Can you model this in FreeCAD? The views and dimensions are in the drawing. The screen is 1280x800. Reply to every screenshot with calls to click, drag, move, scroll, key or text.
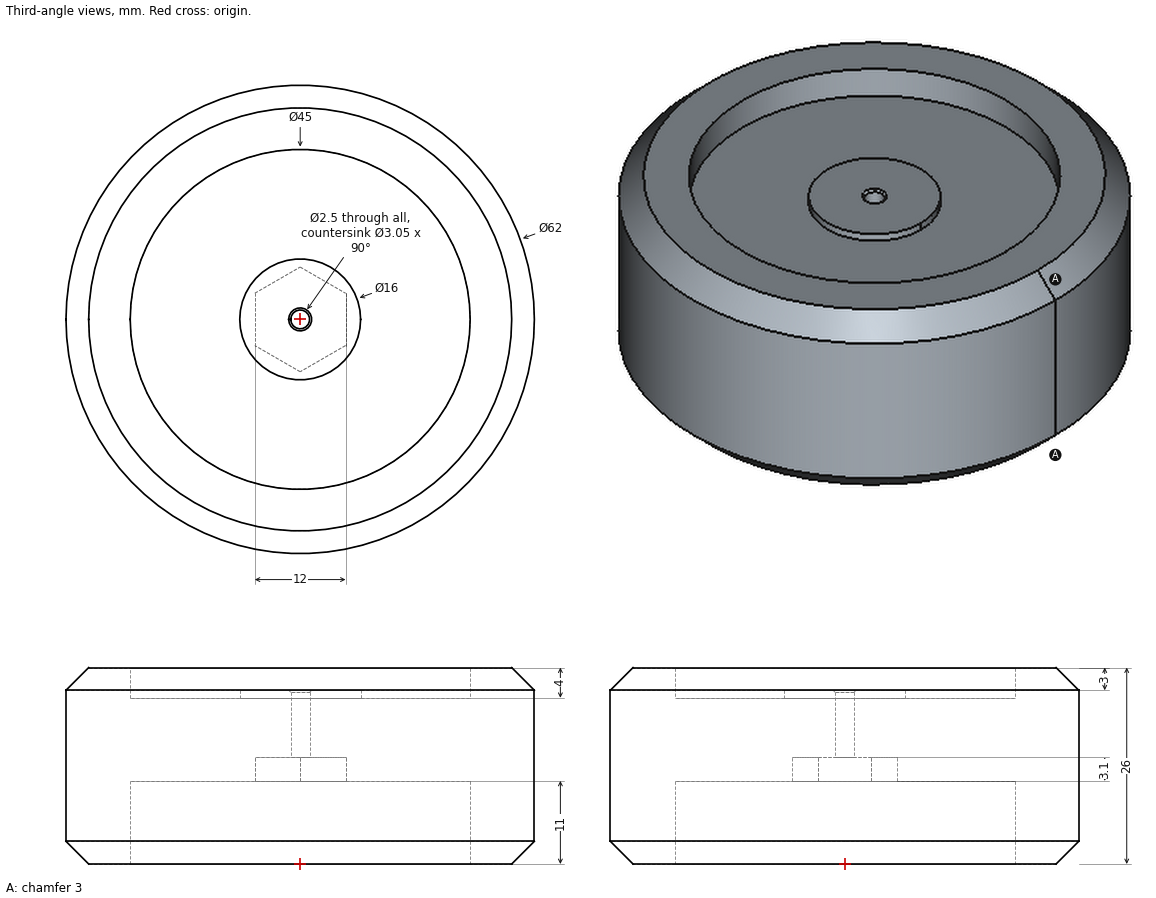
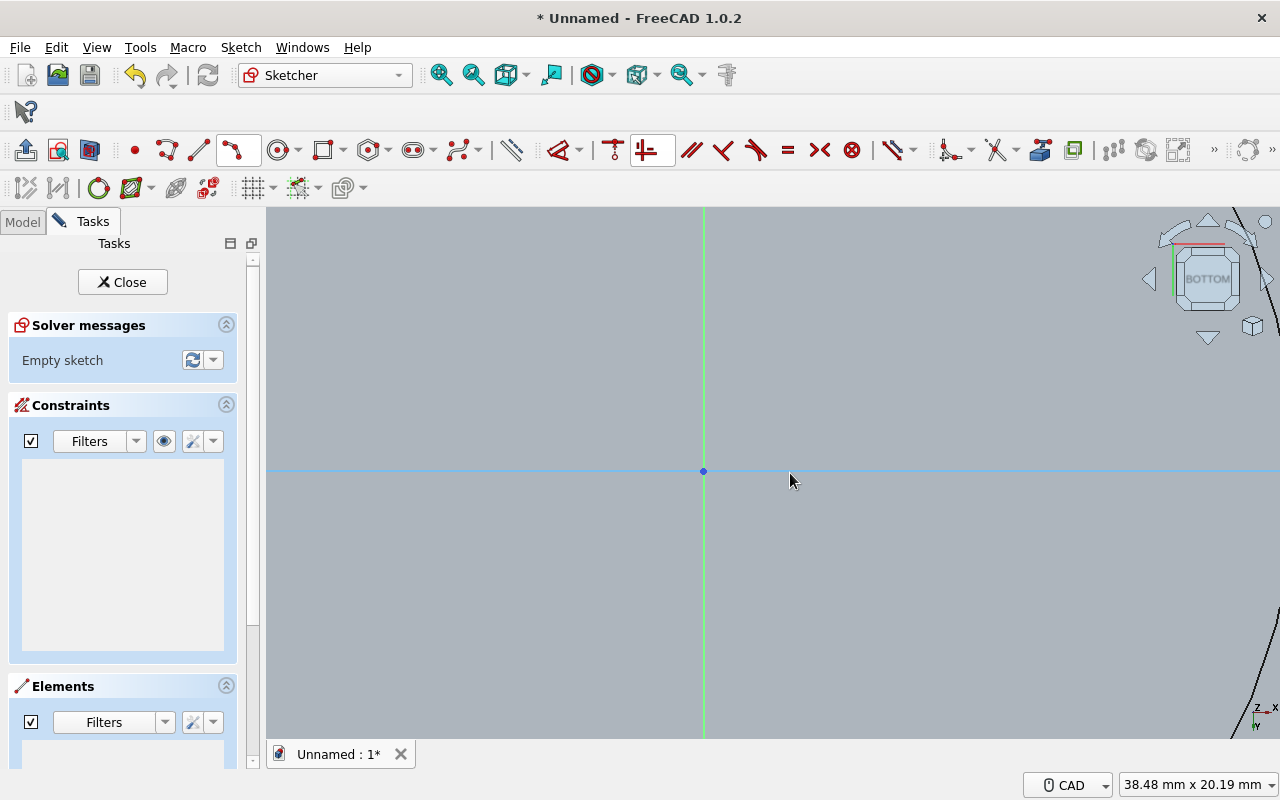
click(368, 150)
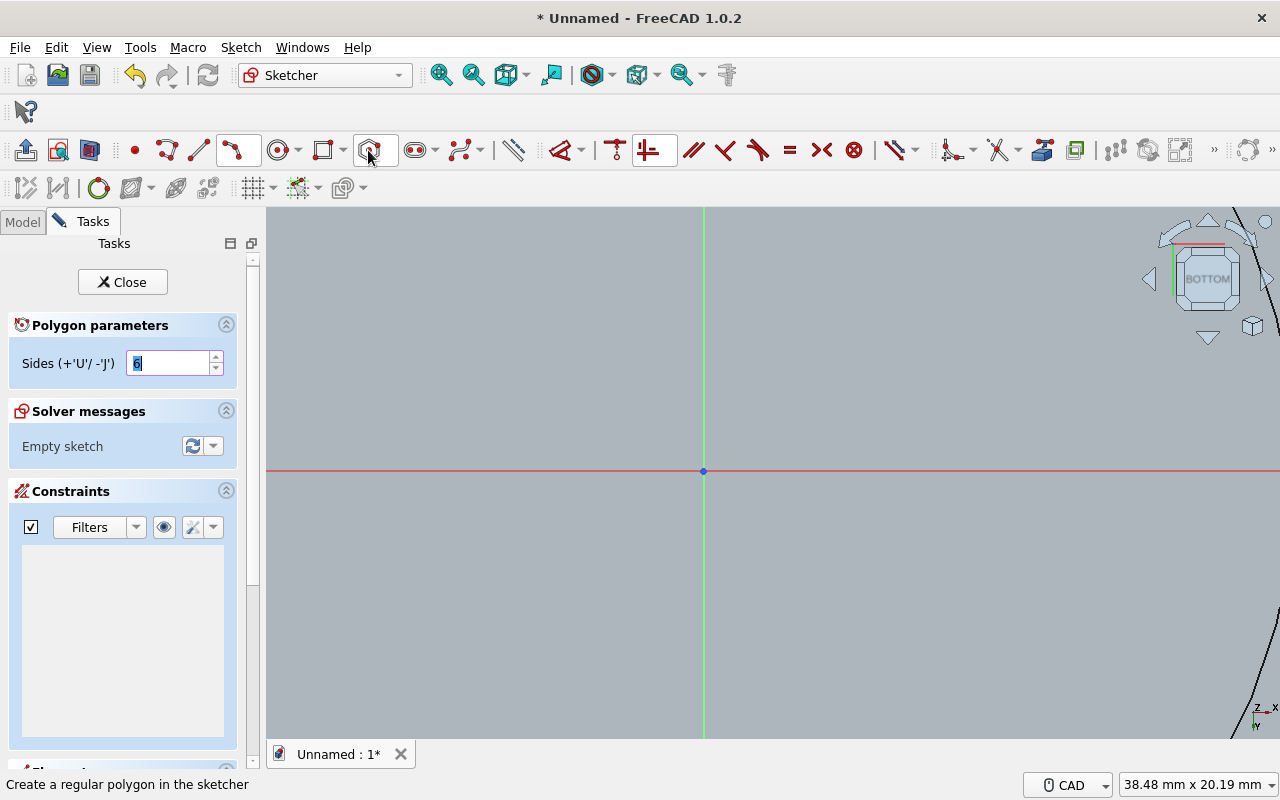
click(704, 471)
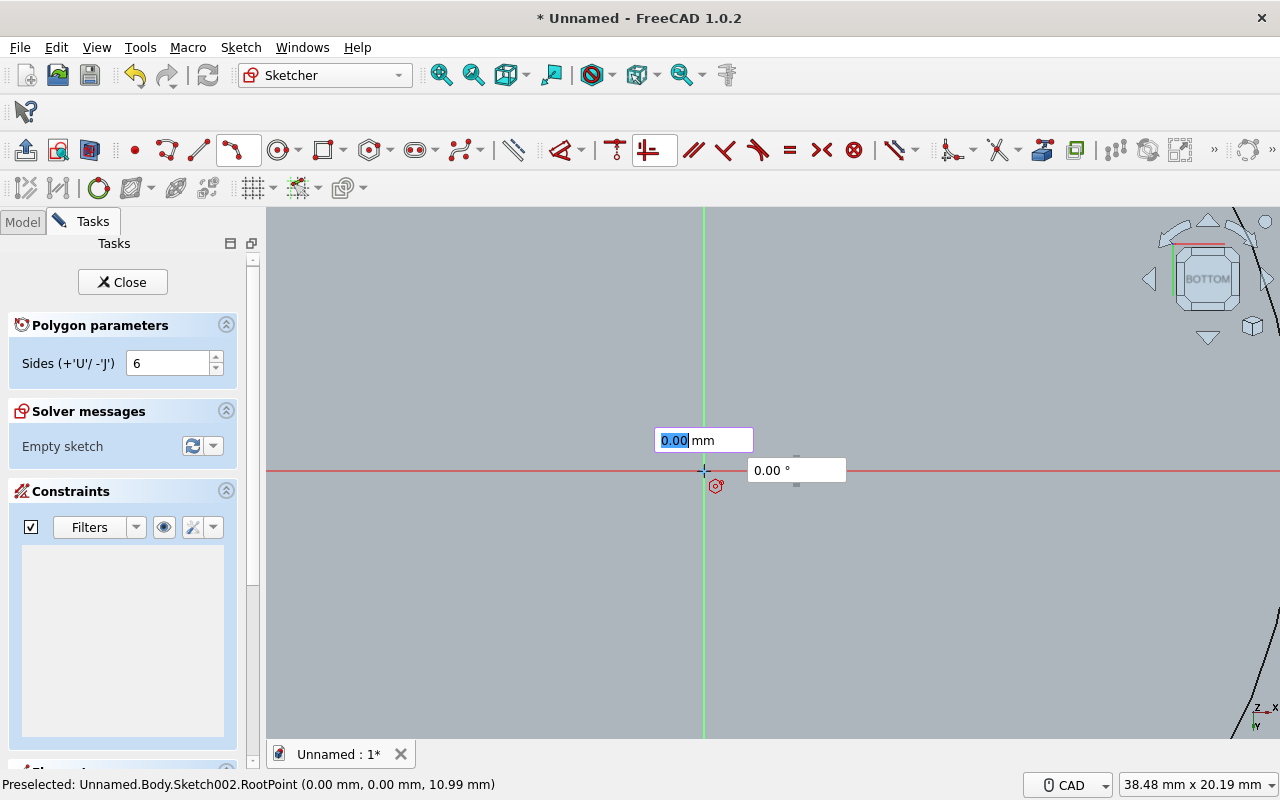
click(704, 654)
right_click(704, 654)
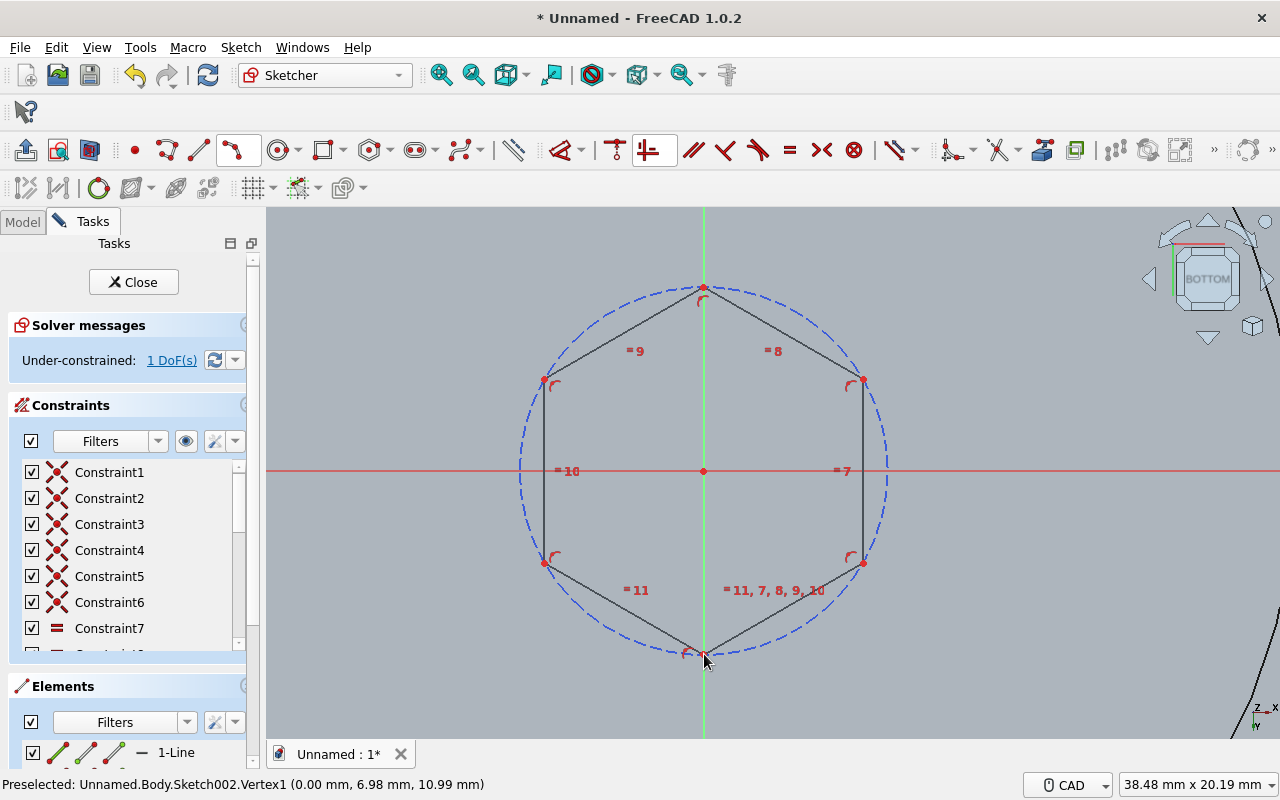
key(d)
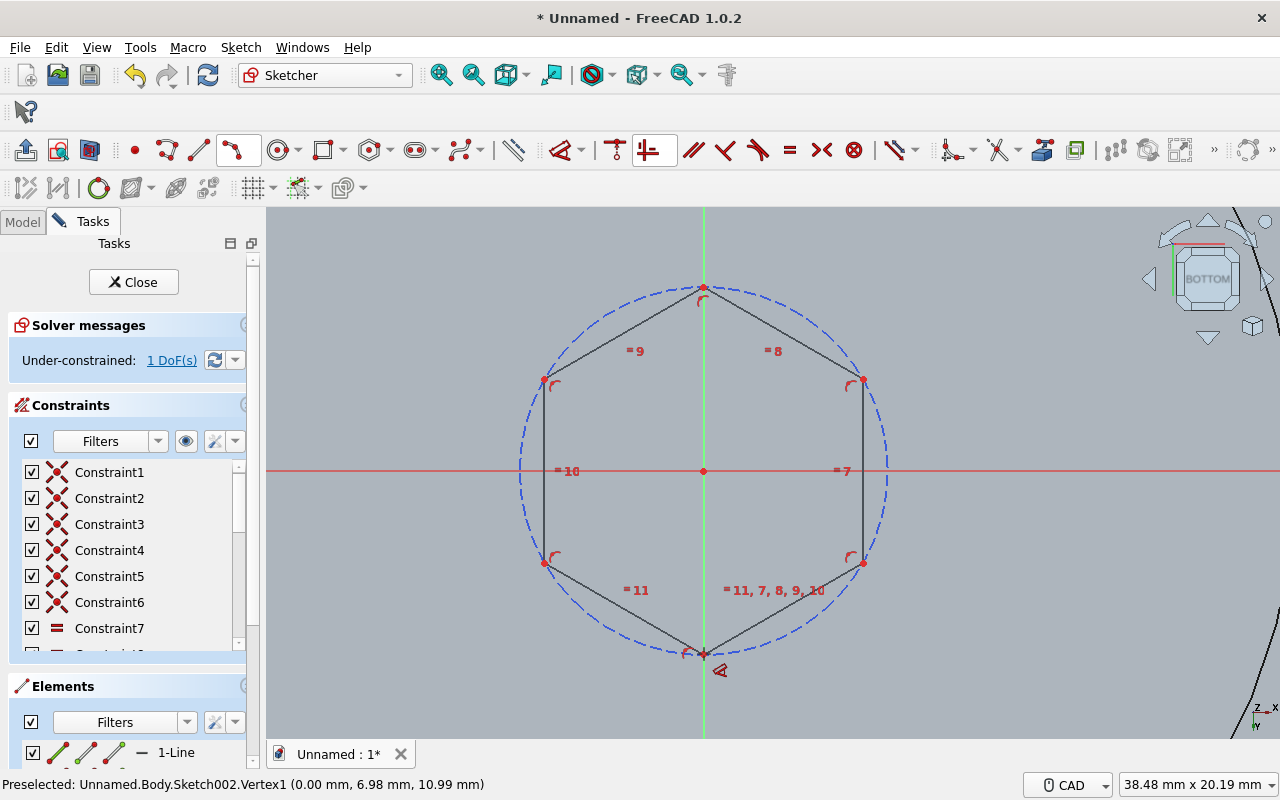
click(544, 379)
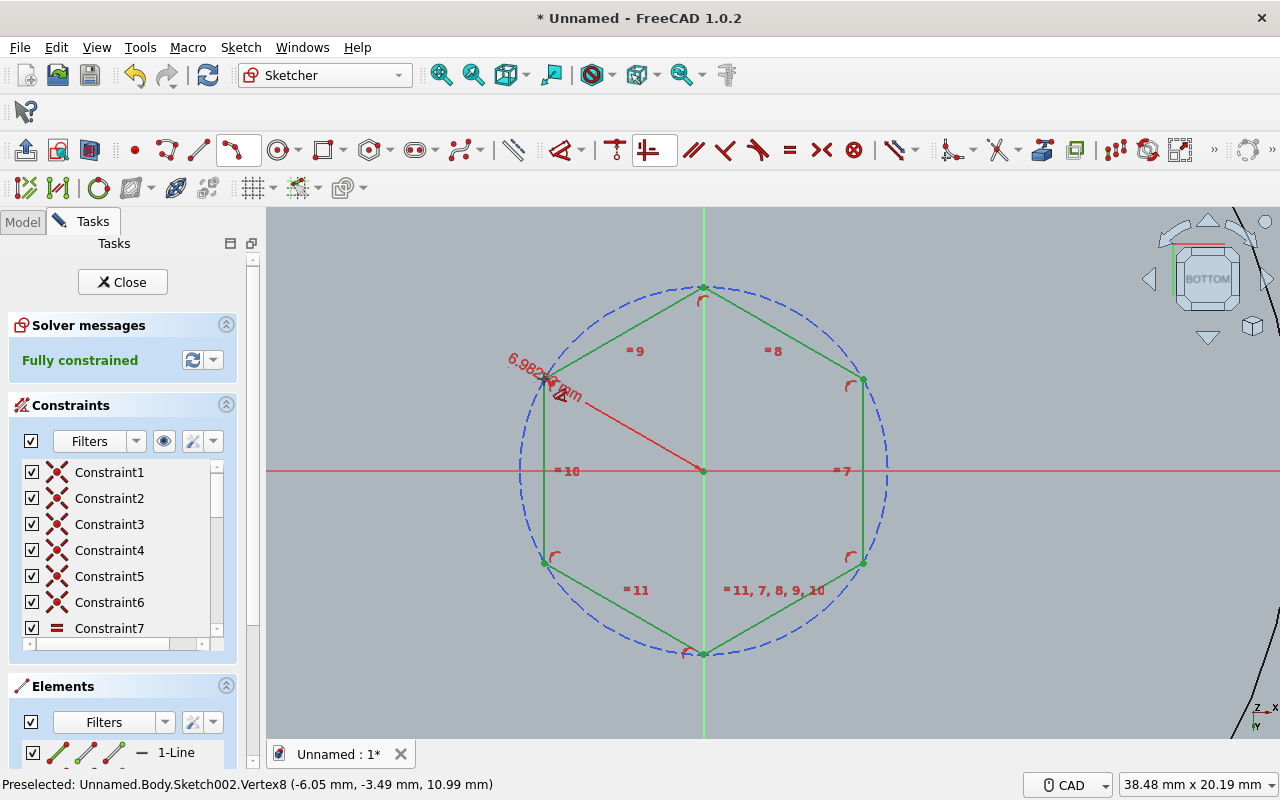
click(863, 563)
click(630, 597)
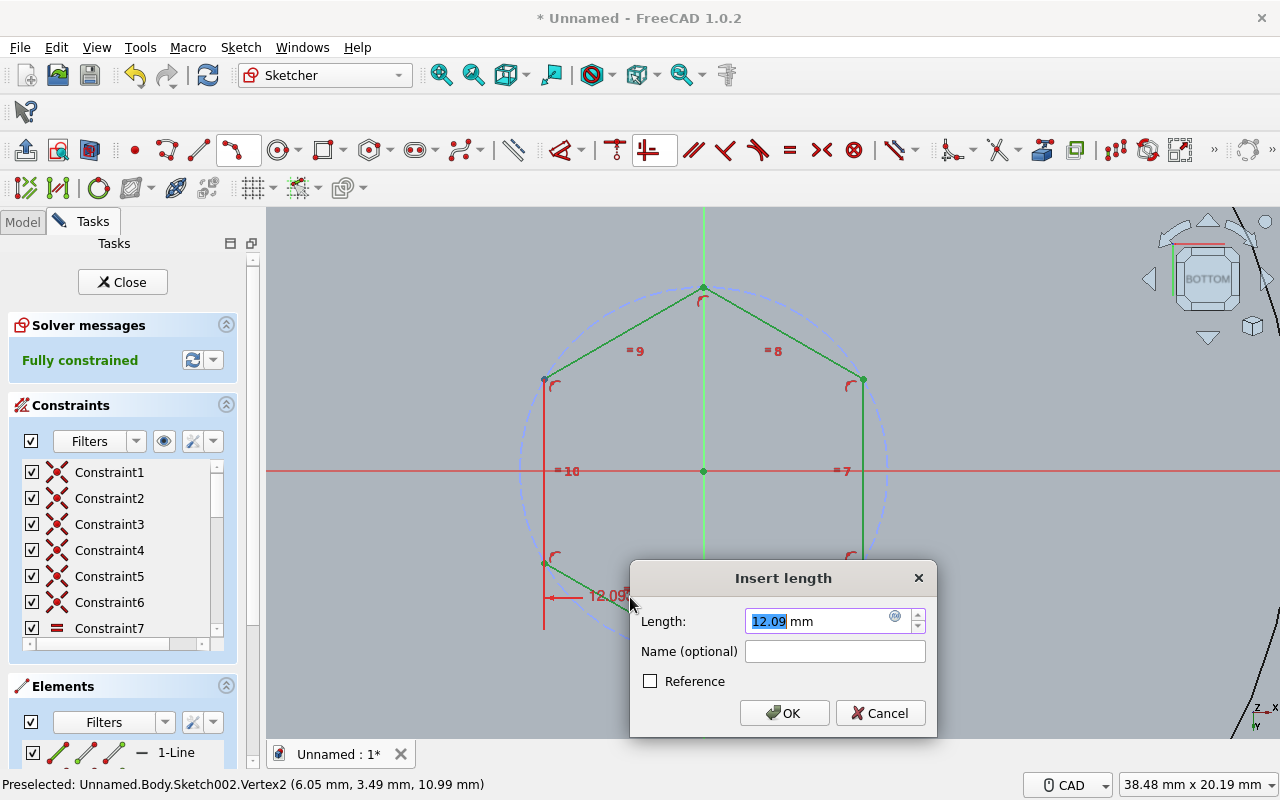
text(12)
key(Return)
key(Escape)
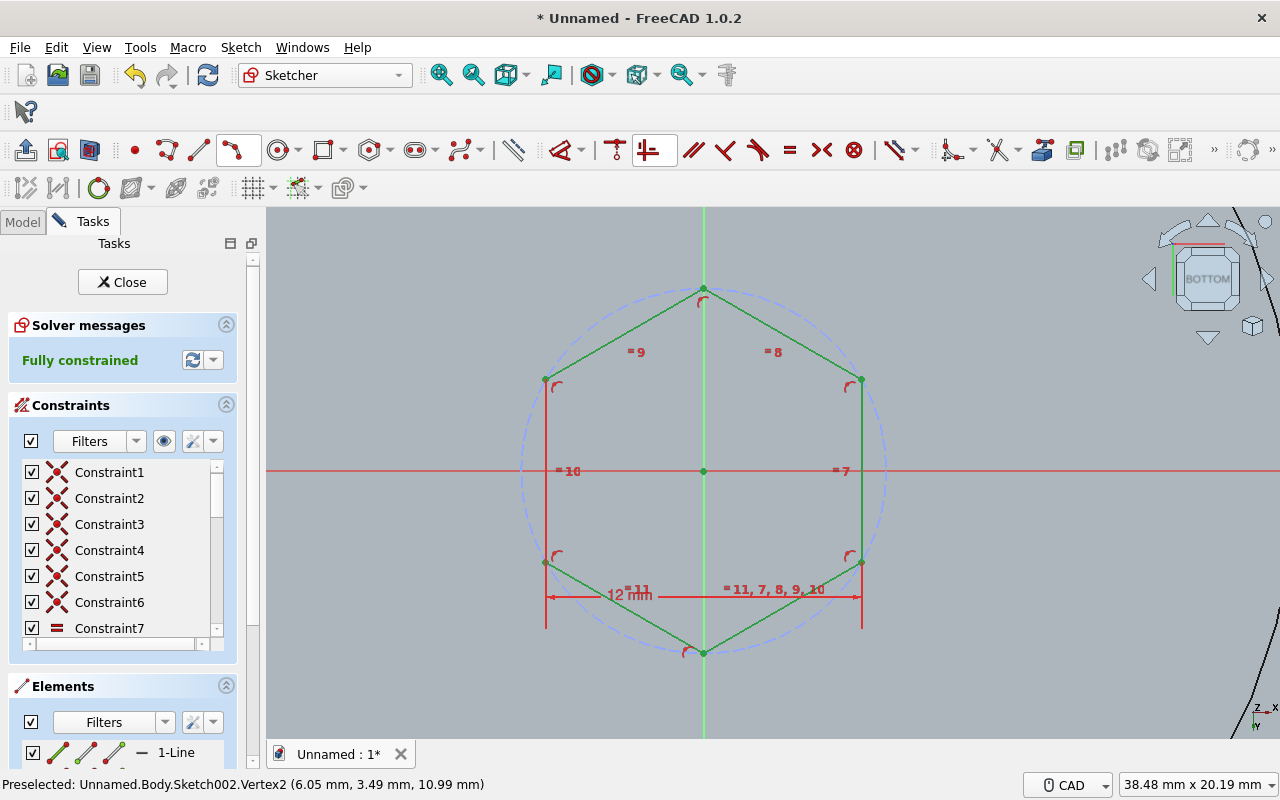
click(123, 282)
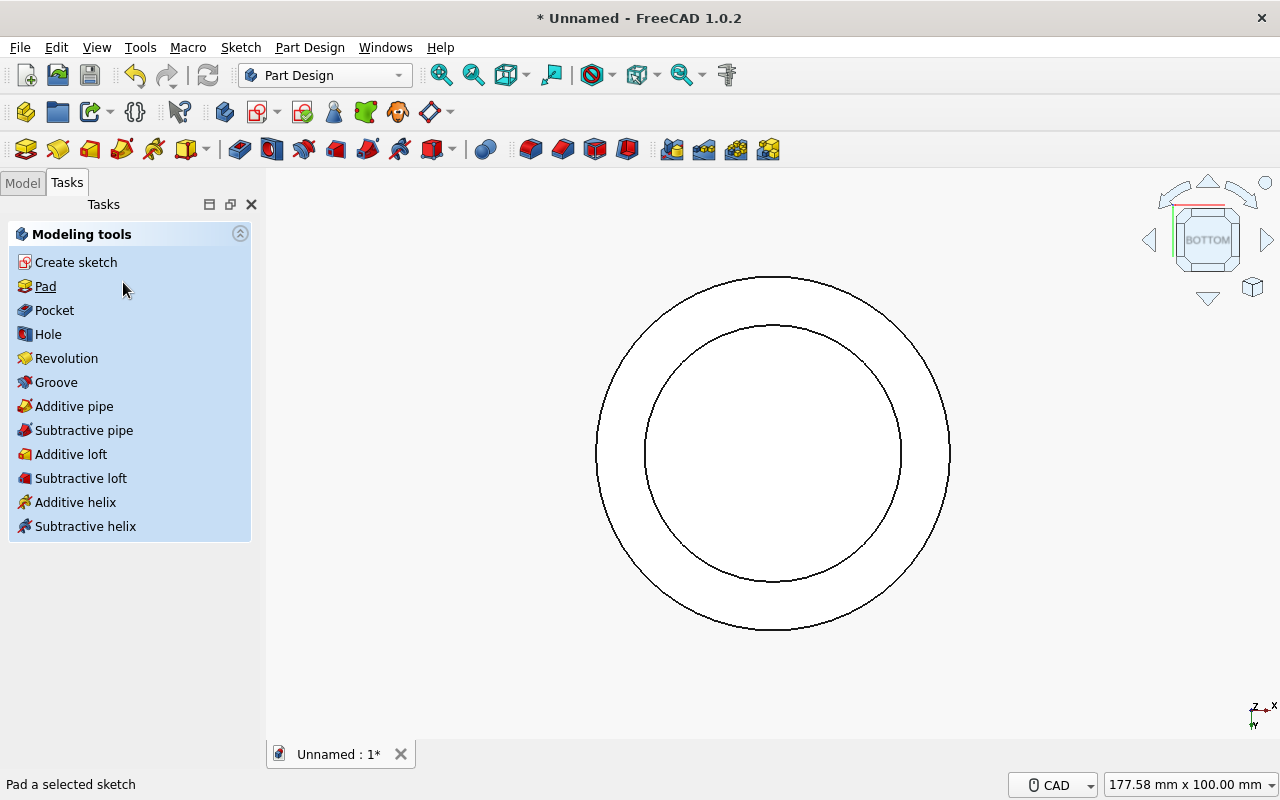
click(240, 150)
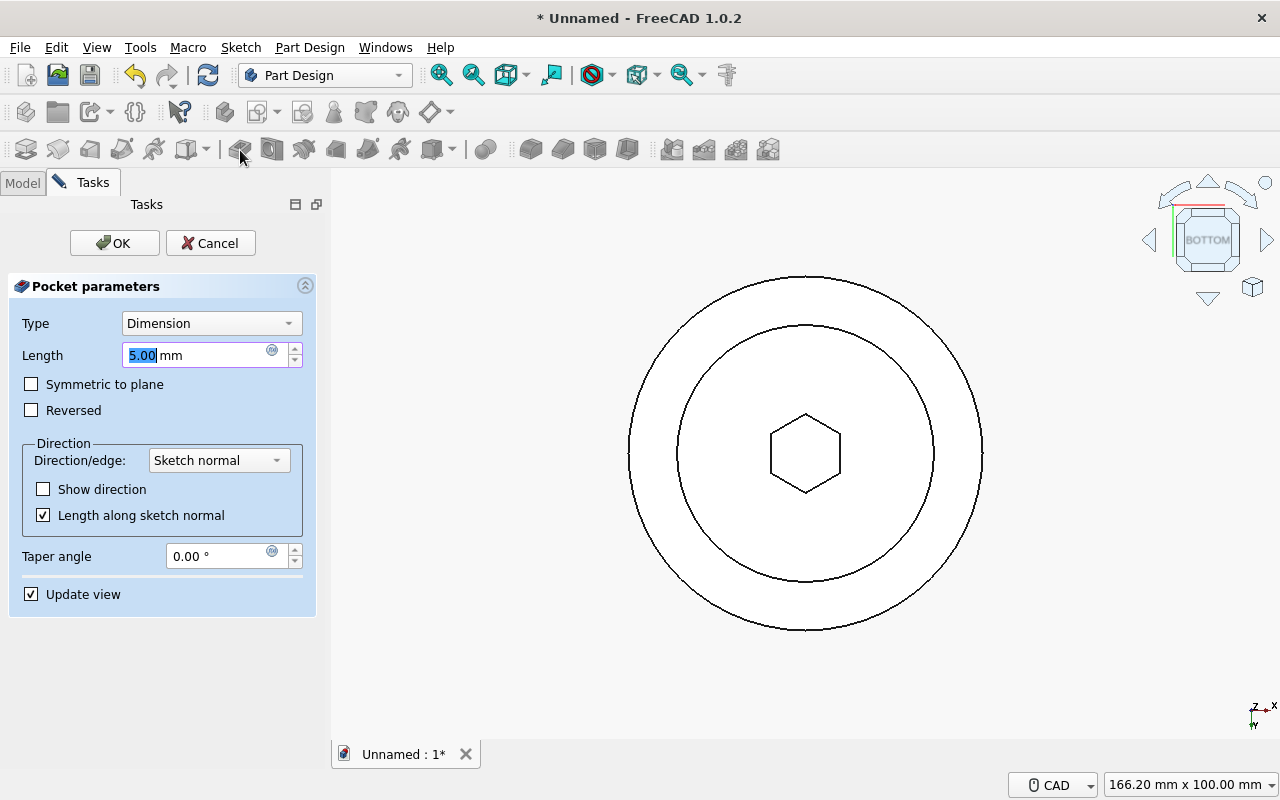
text(3.1)
key(Tab)